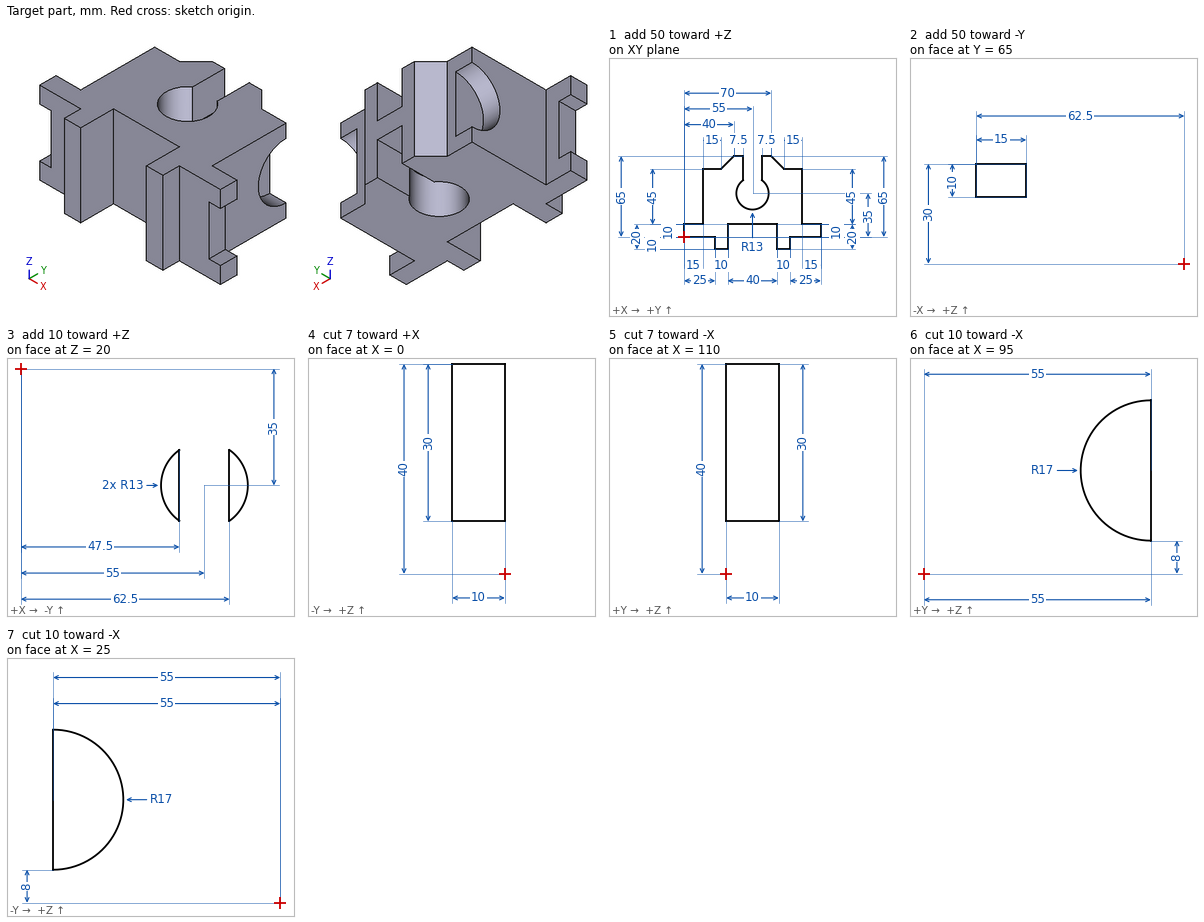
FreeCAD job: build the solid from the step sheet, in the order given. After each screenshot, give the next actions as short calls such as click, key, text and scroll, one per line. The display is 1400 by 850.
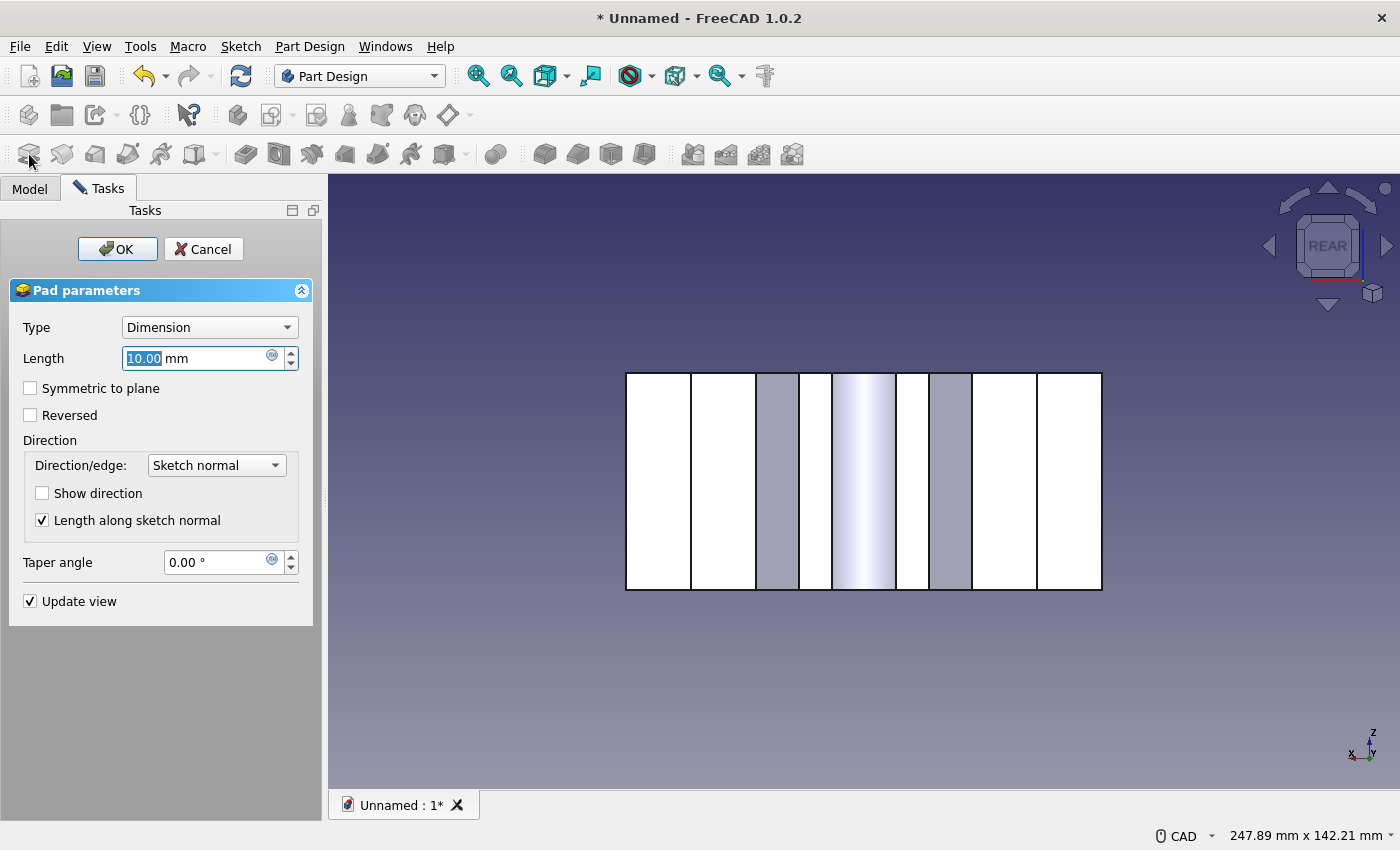
text(50)
key(Tab)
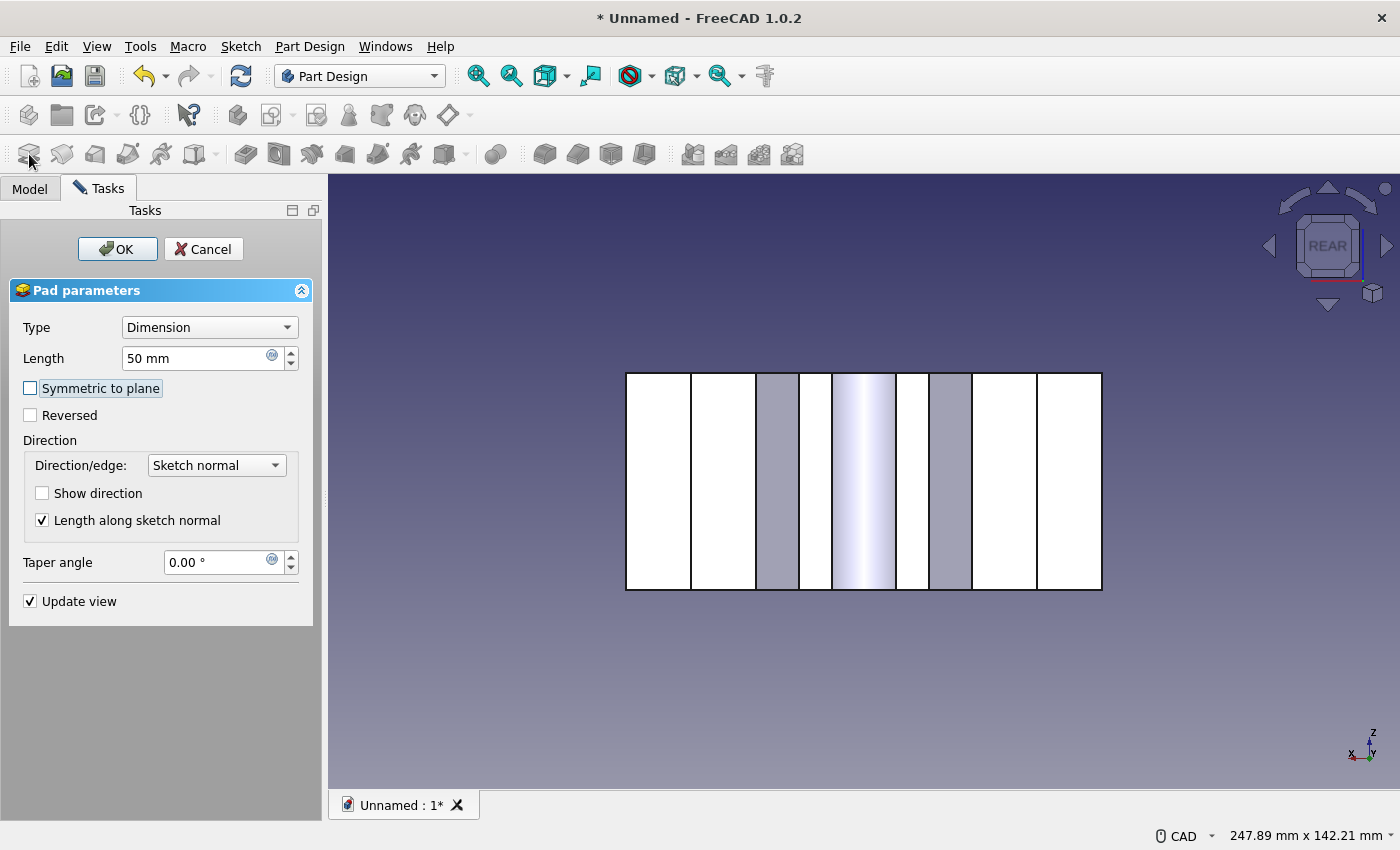
click(31, 415)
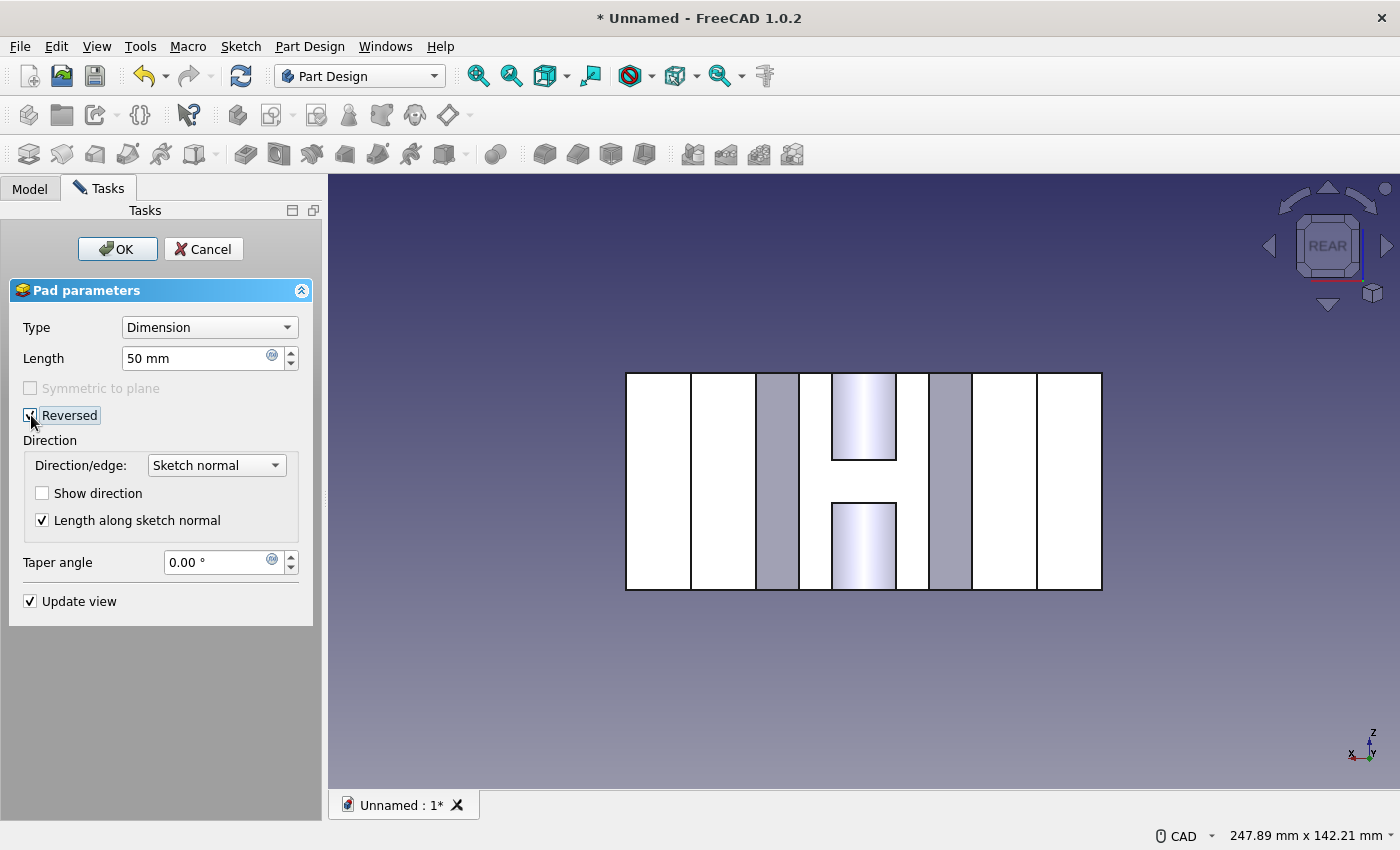
click(118, 249)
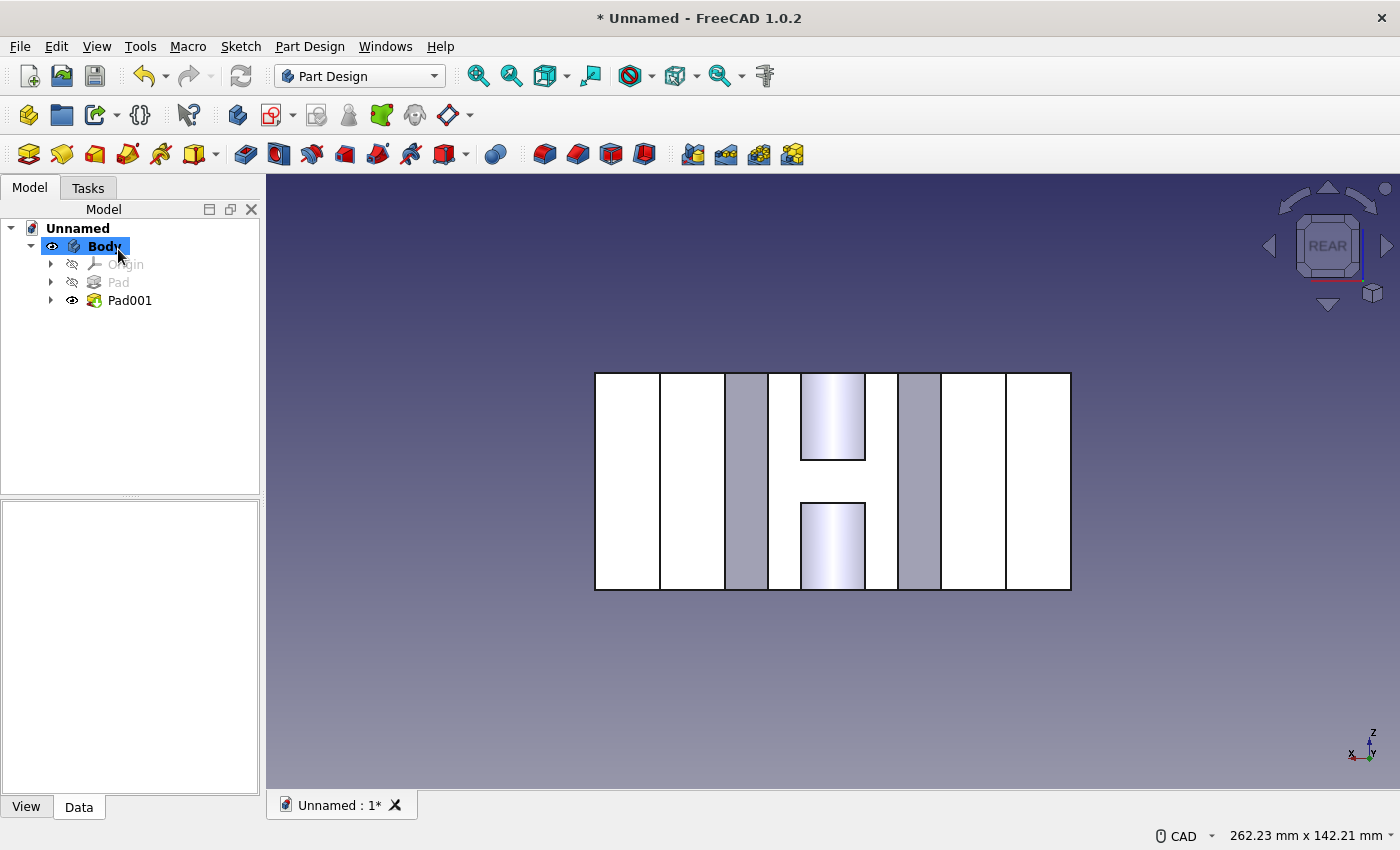
click(479, 76)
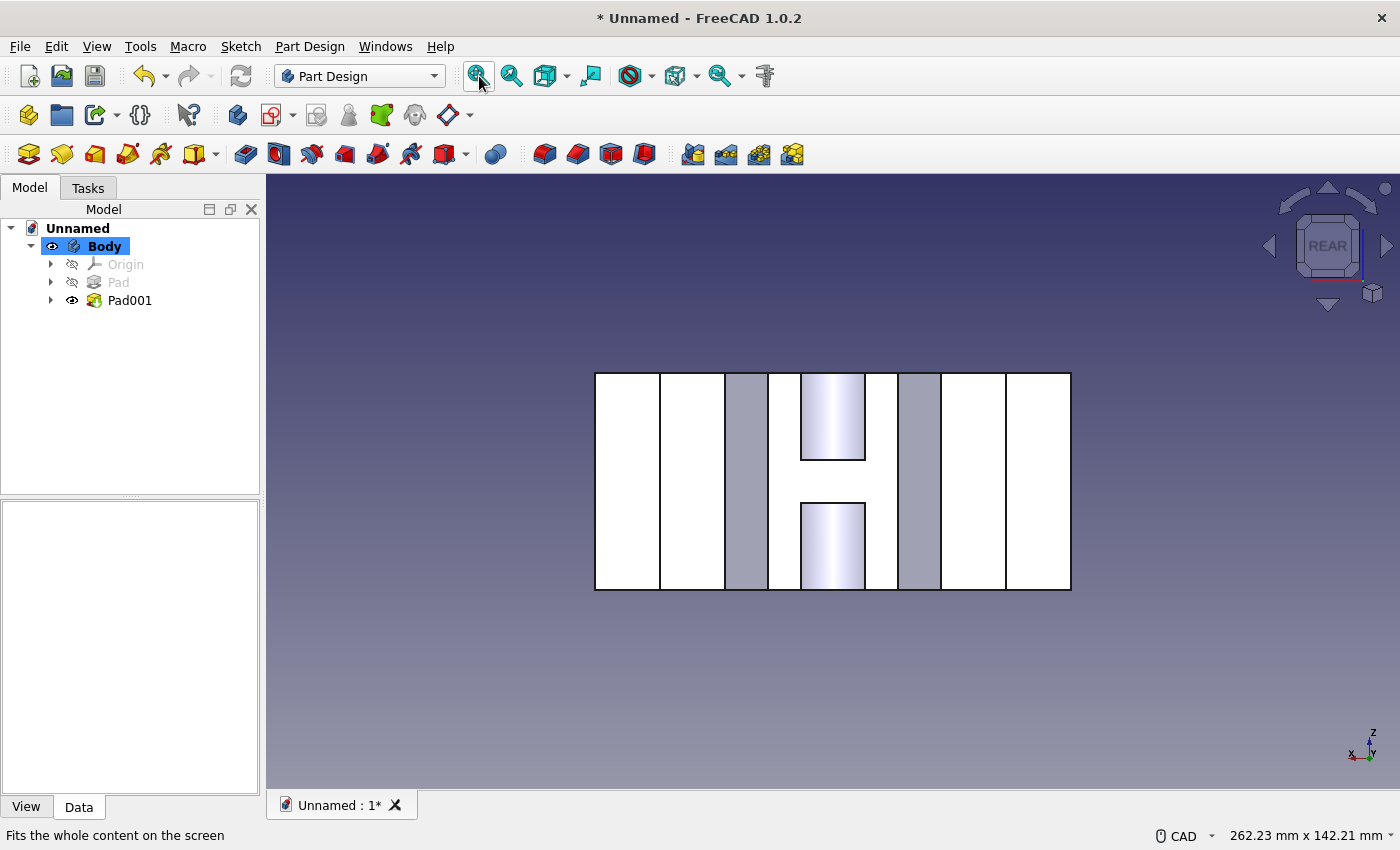
key(5)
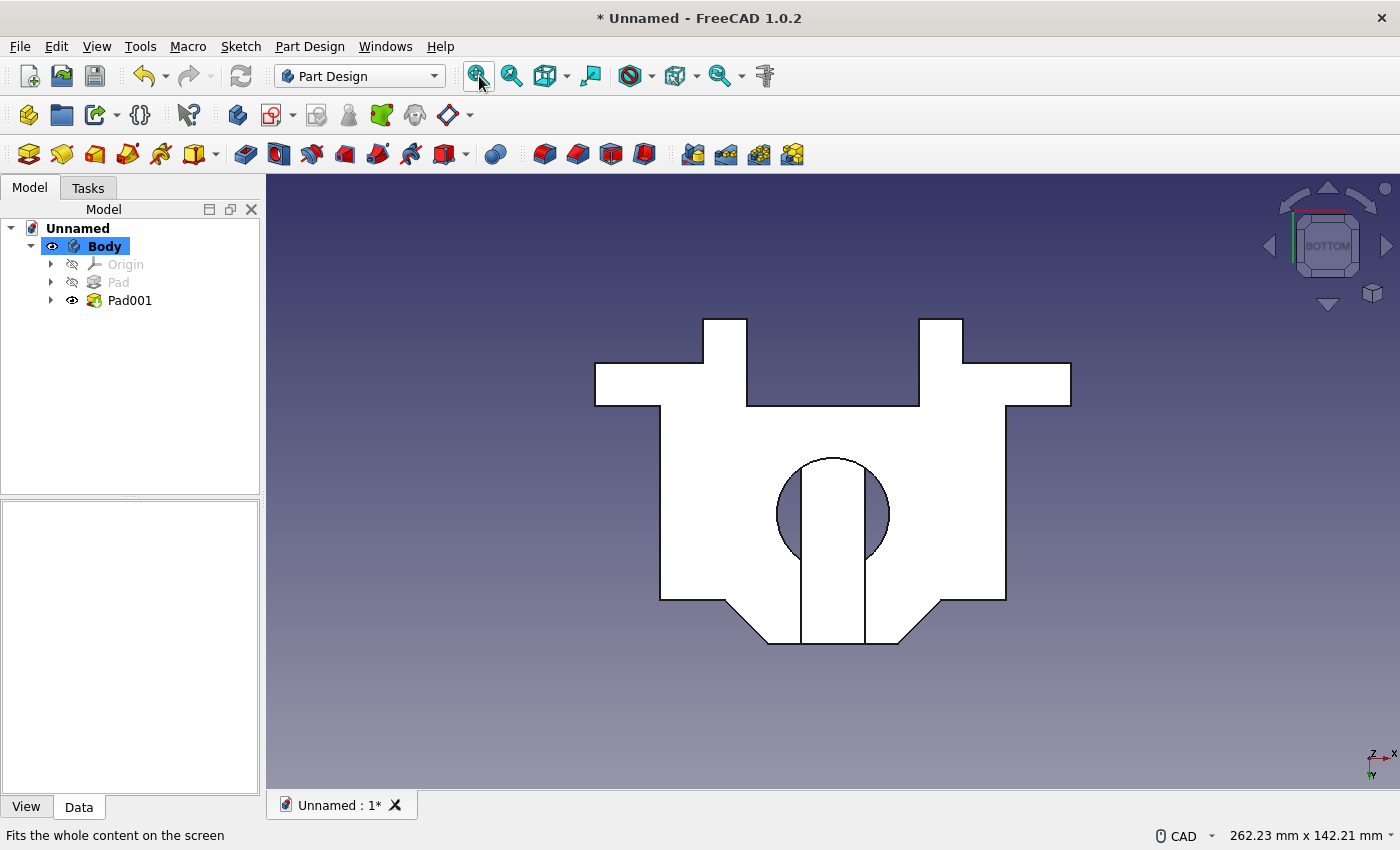
click(833, 603)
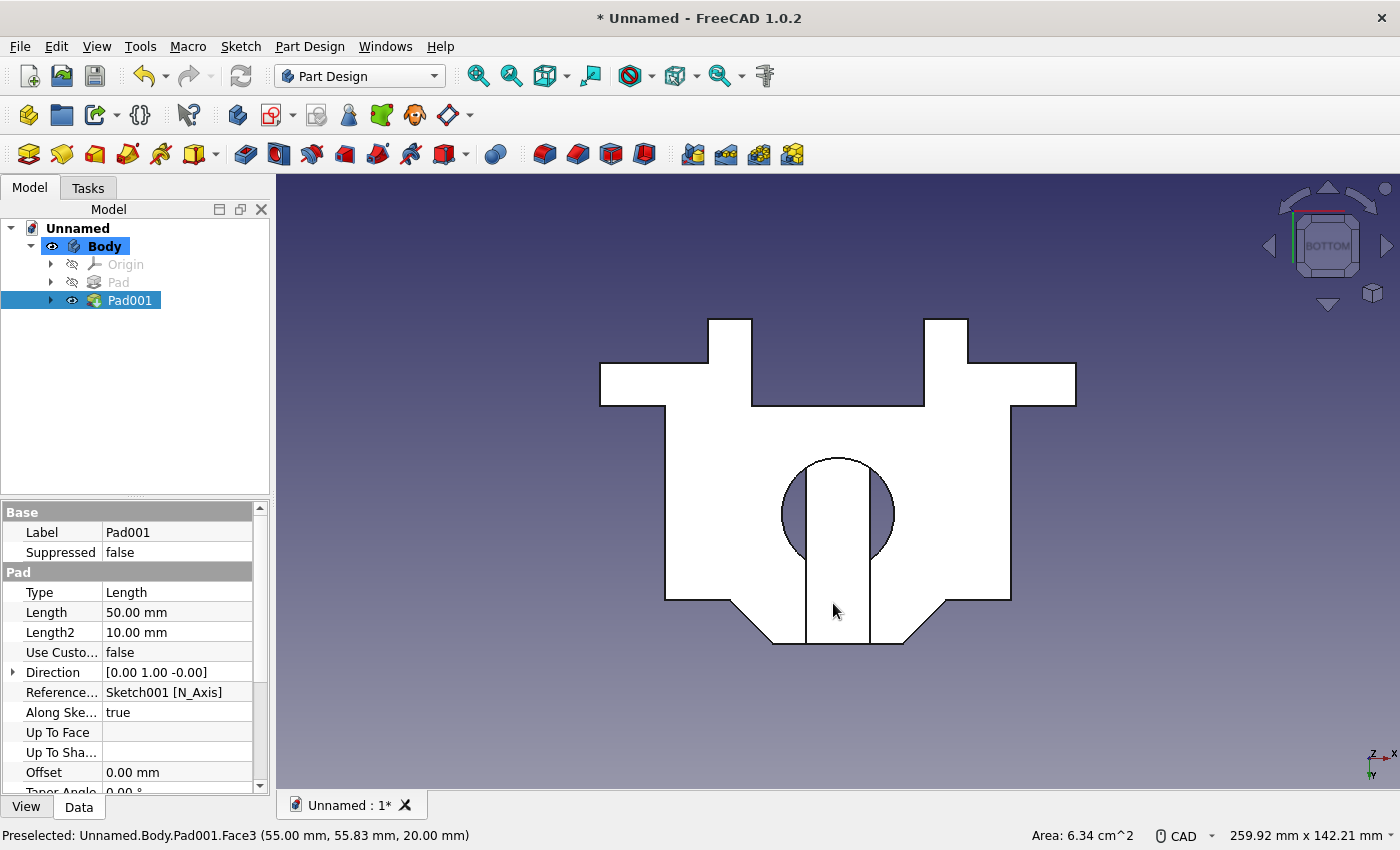
click(270, 116)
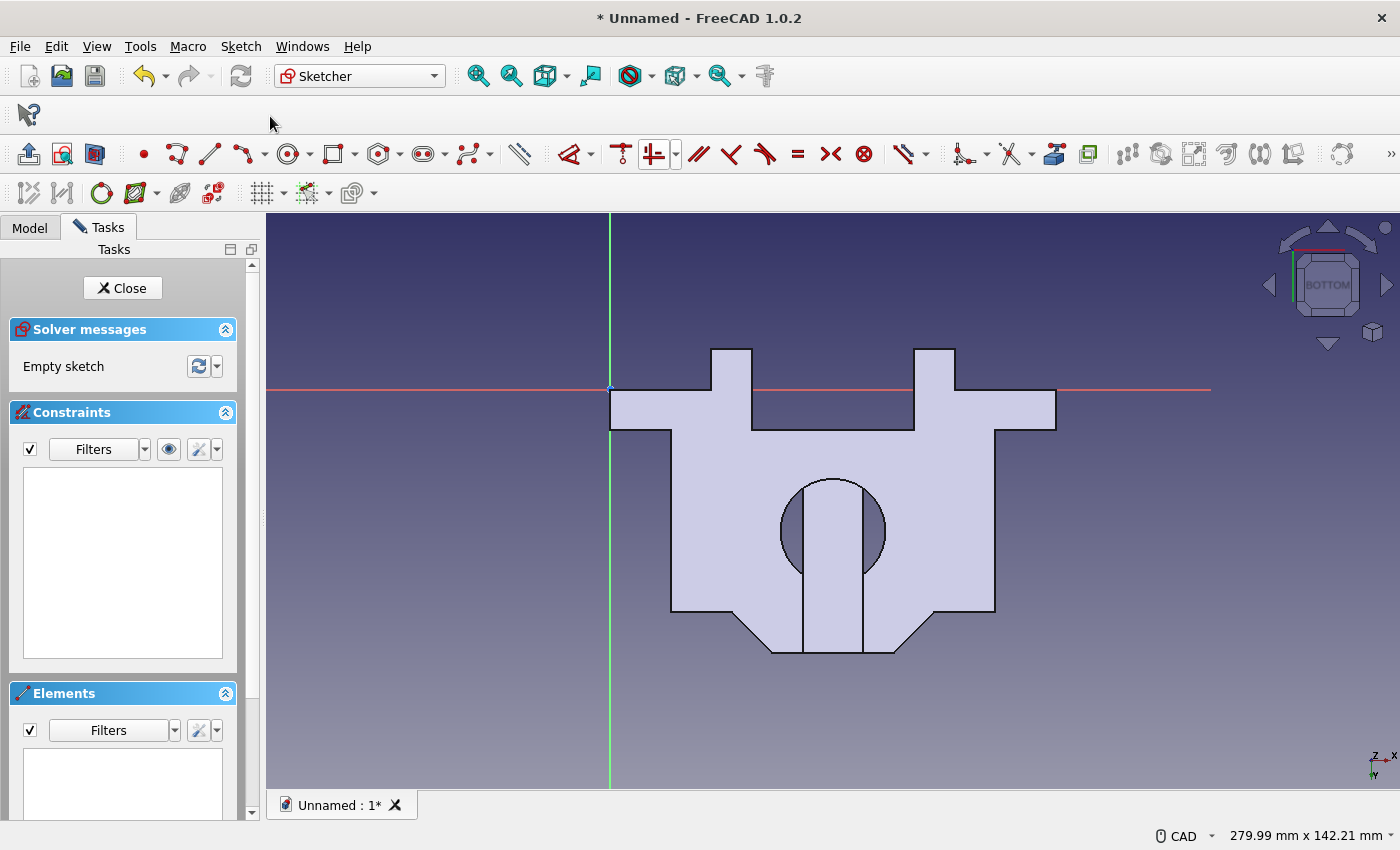
scroll(855, 541, up, 7)